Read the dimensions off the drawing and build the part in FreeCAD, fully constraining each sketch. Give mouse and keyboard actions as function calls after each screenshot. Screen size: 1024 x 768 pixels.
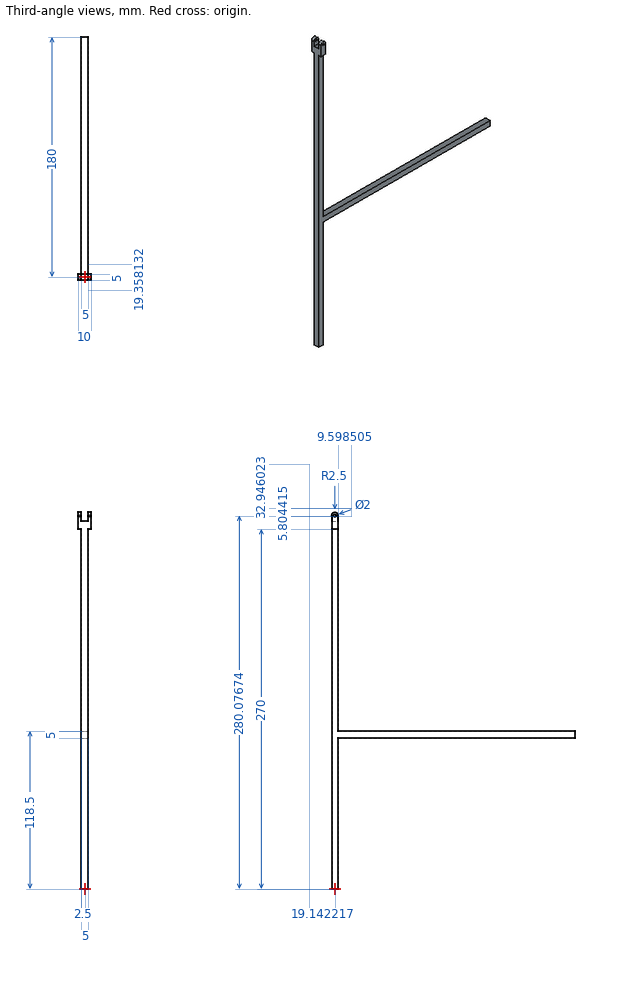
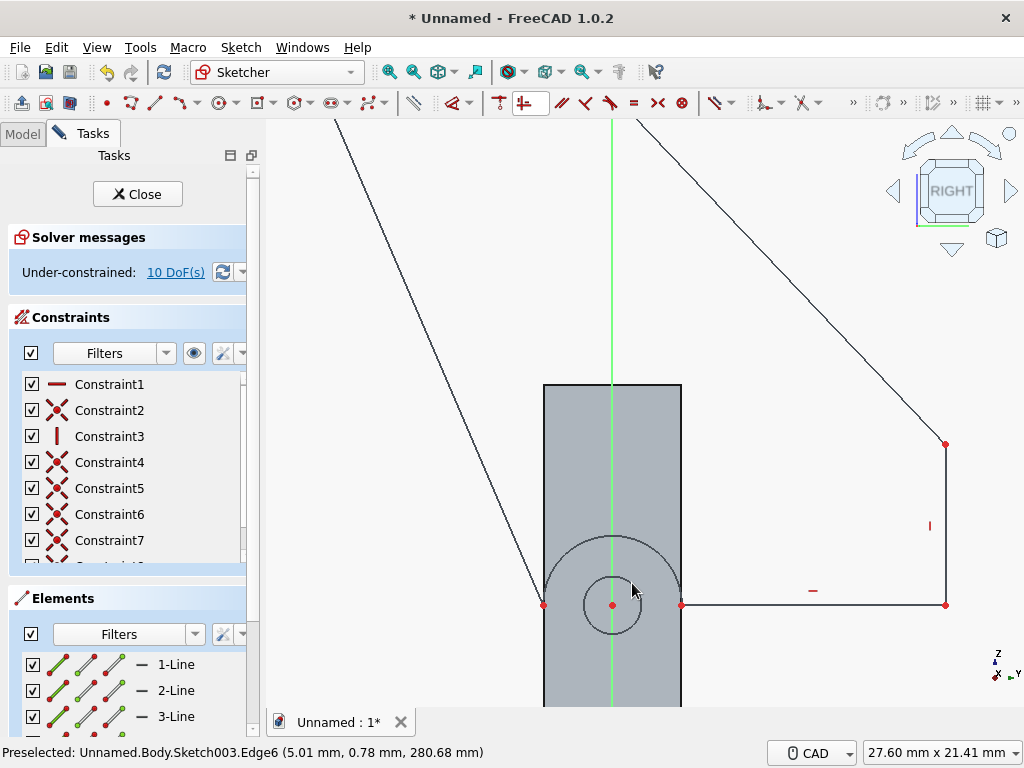
click(613, 605)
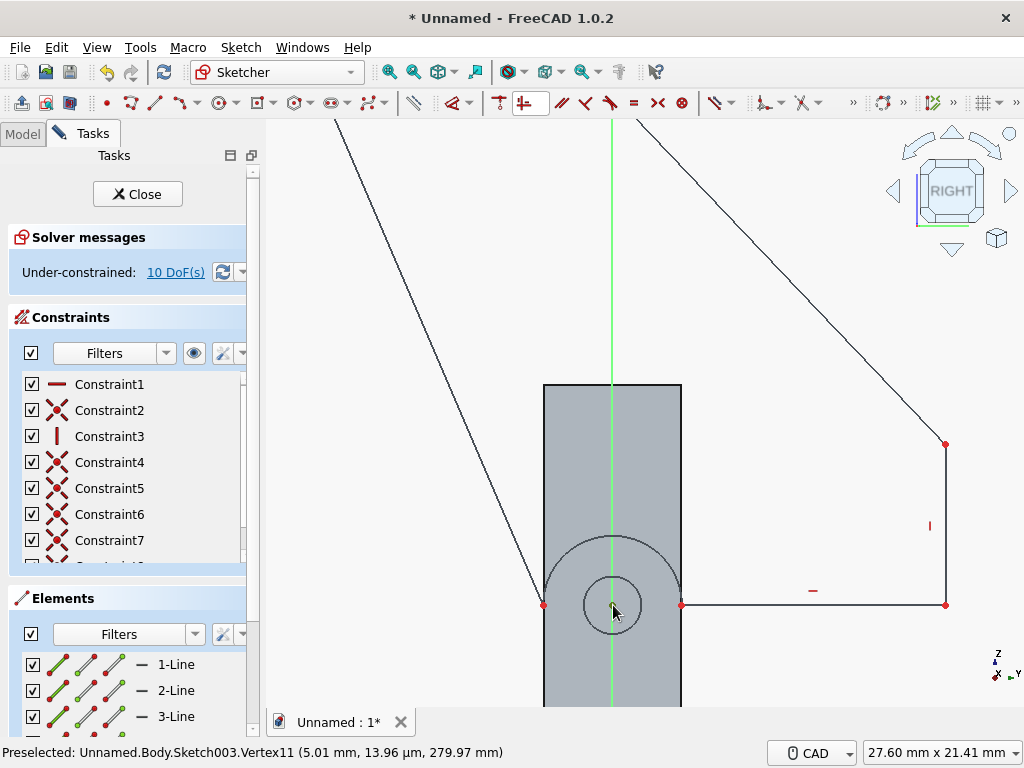
click(612, 489)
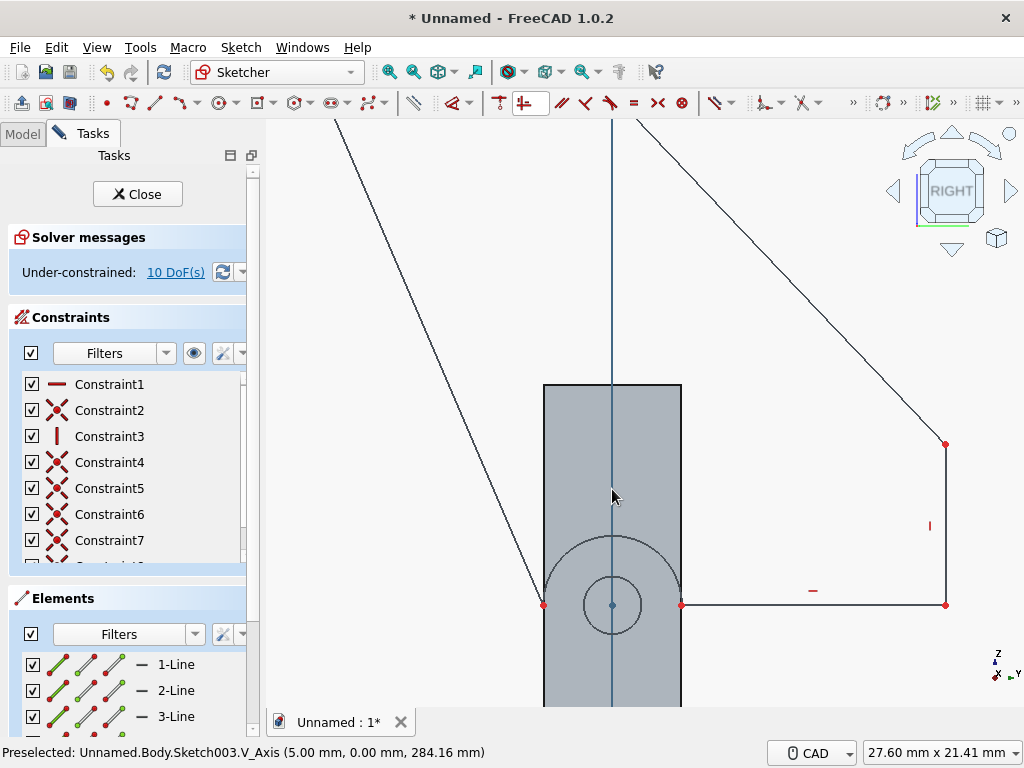
click(500, 104)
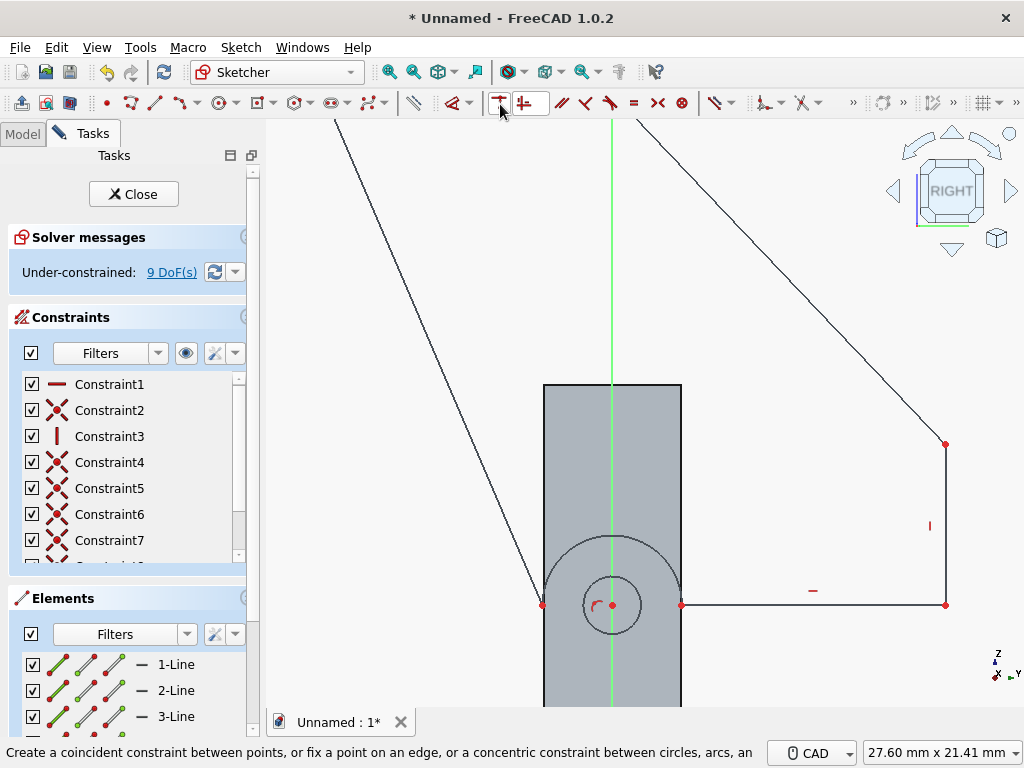
click(452, 104)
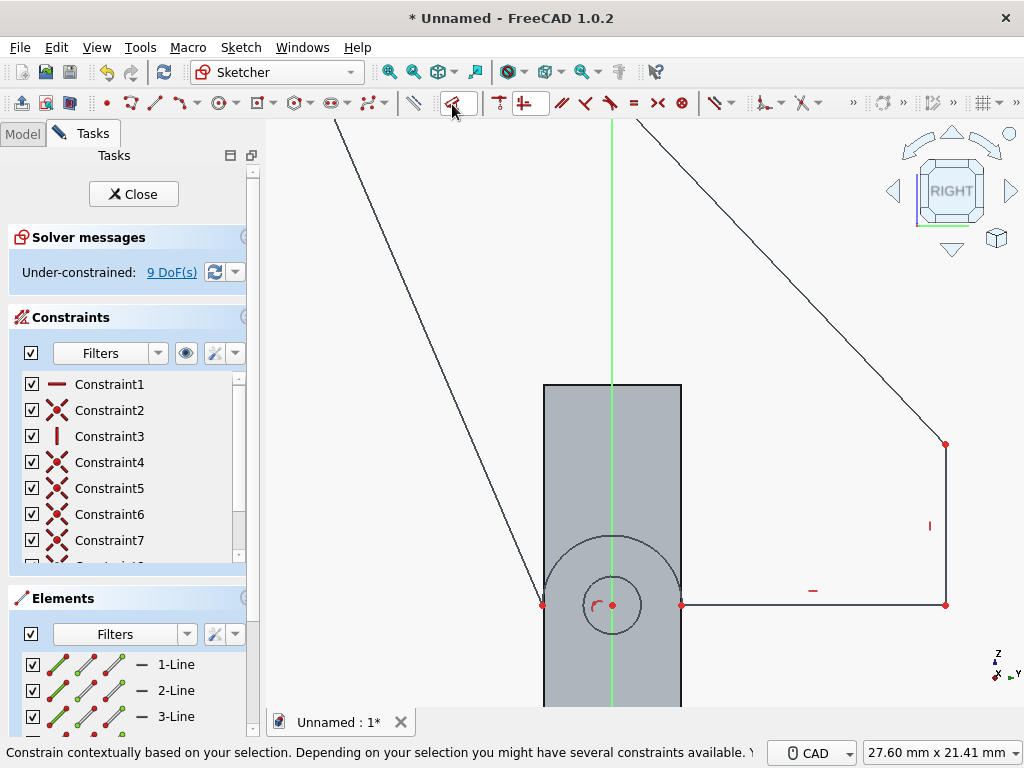
click(653, 549)
click(672, 523)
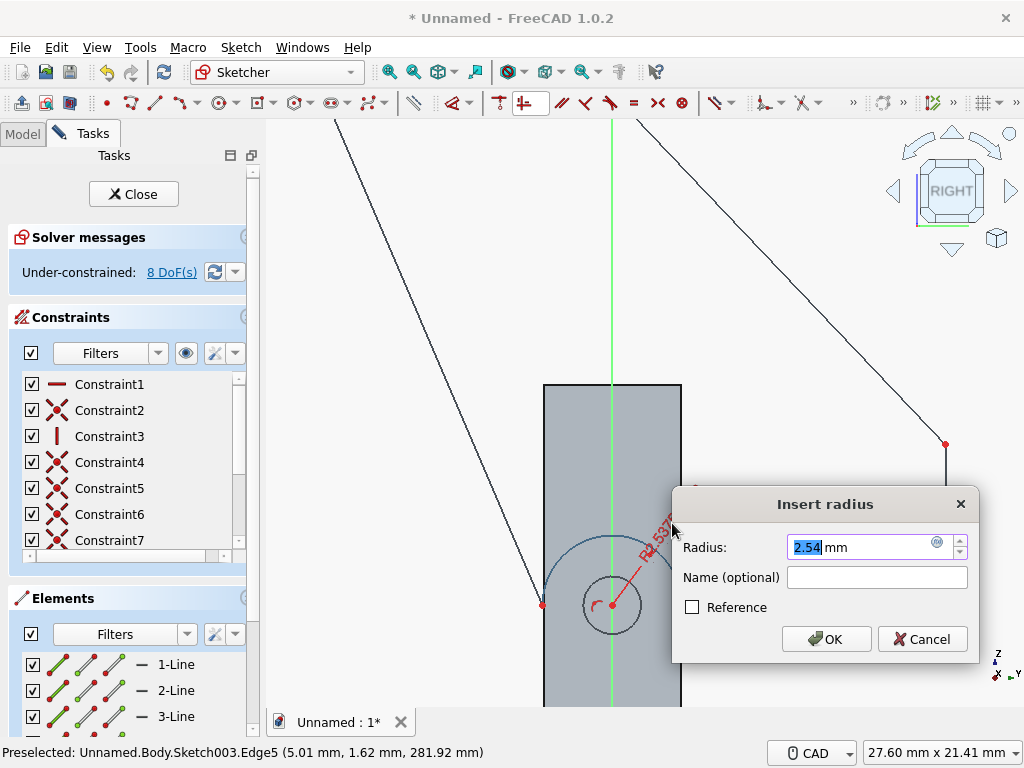
text(2.5)
key(Return)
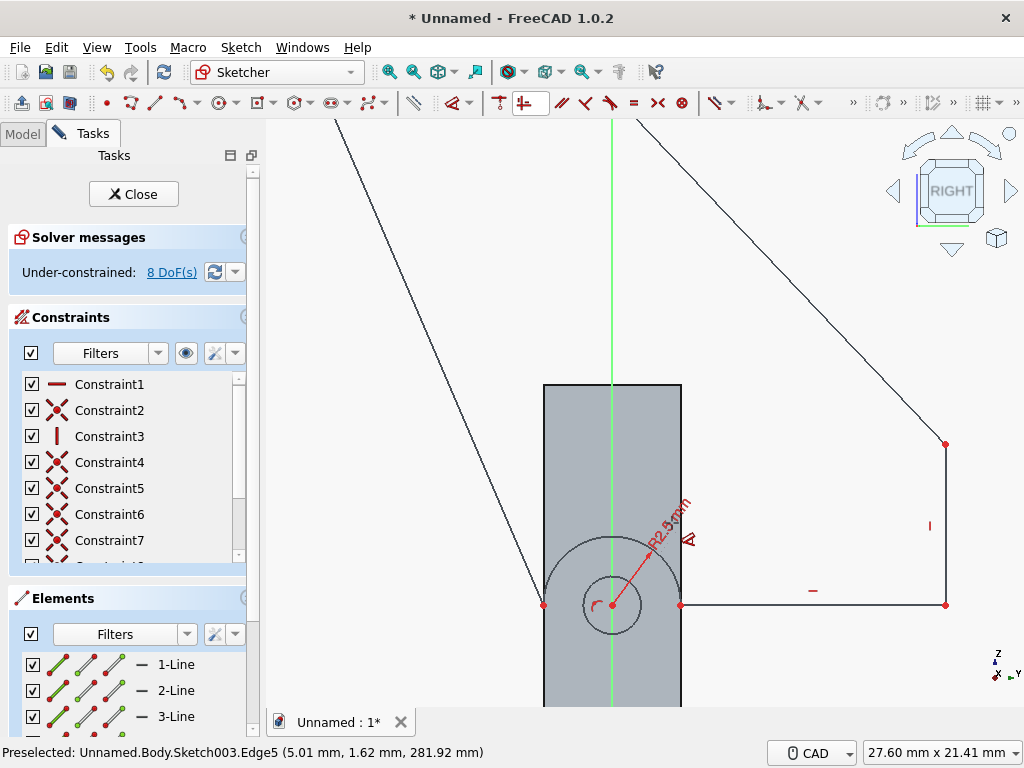
click(632, 585)
click(671, 617)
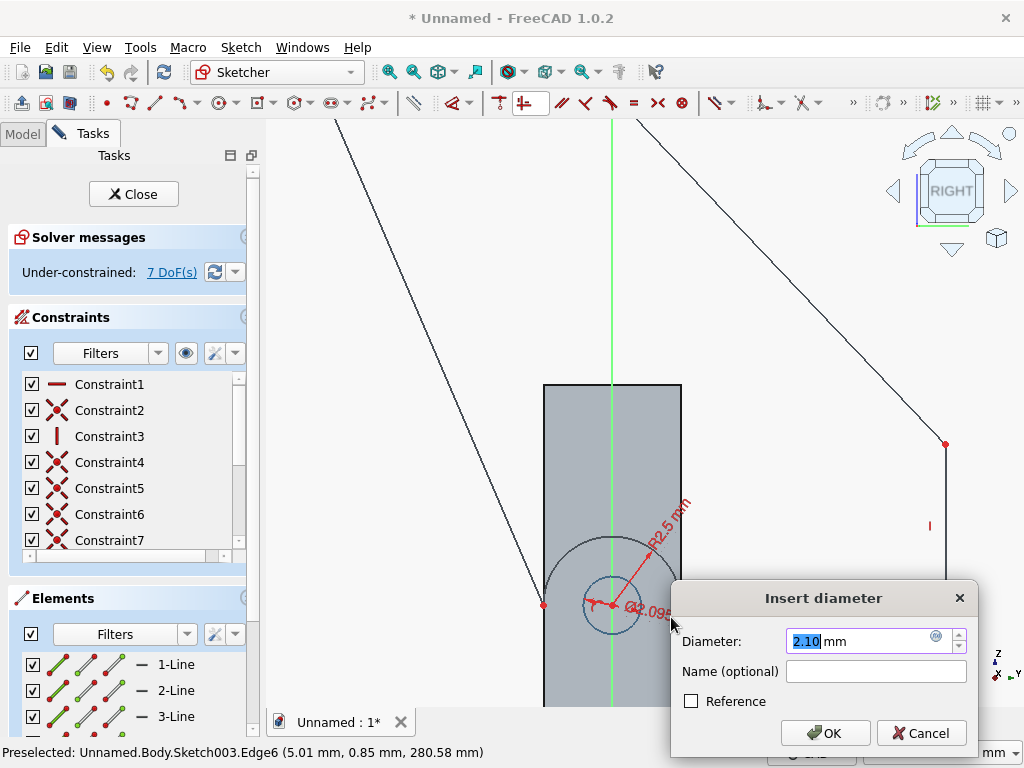
text(2)
key(Return)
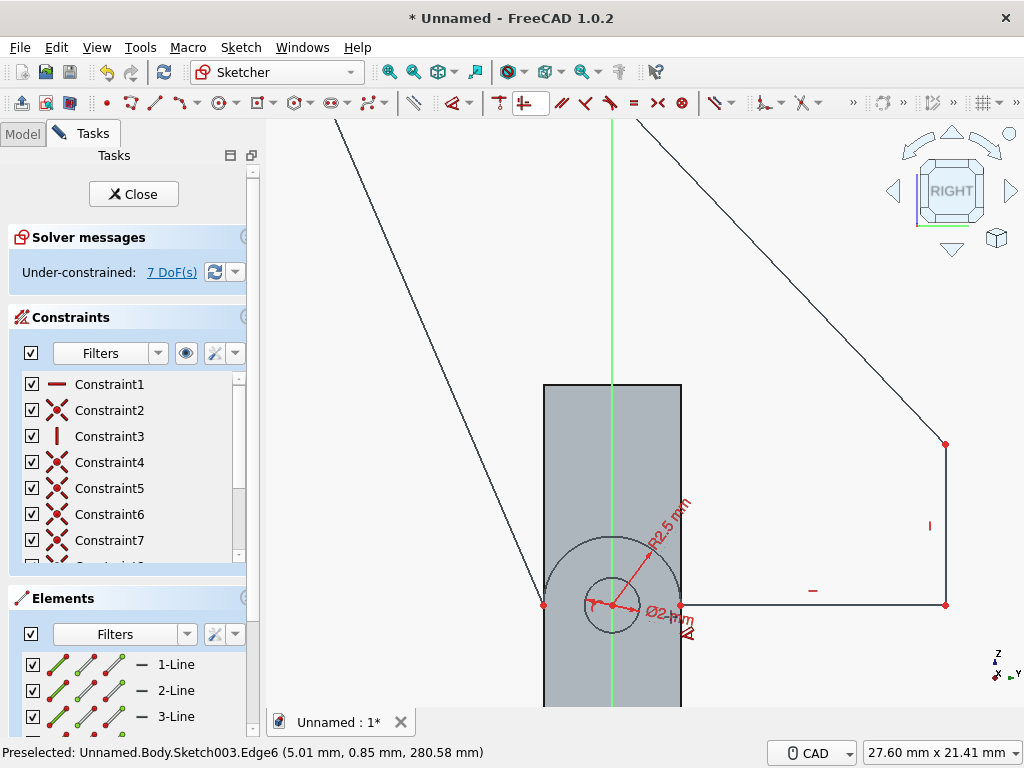
click(760, 605)
click(770, 639)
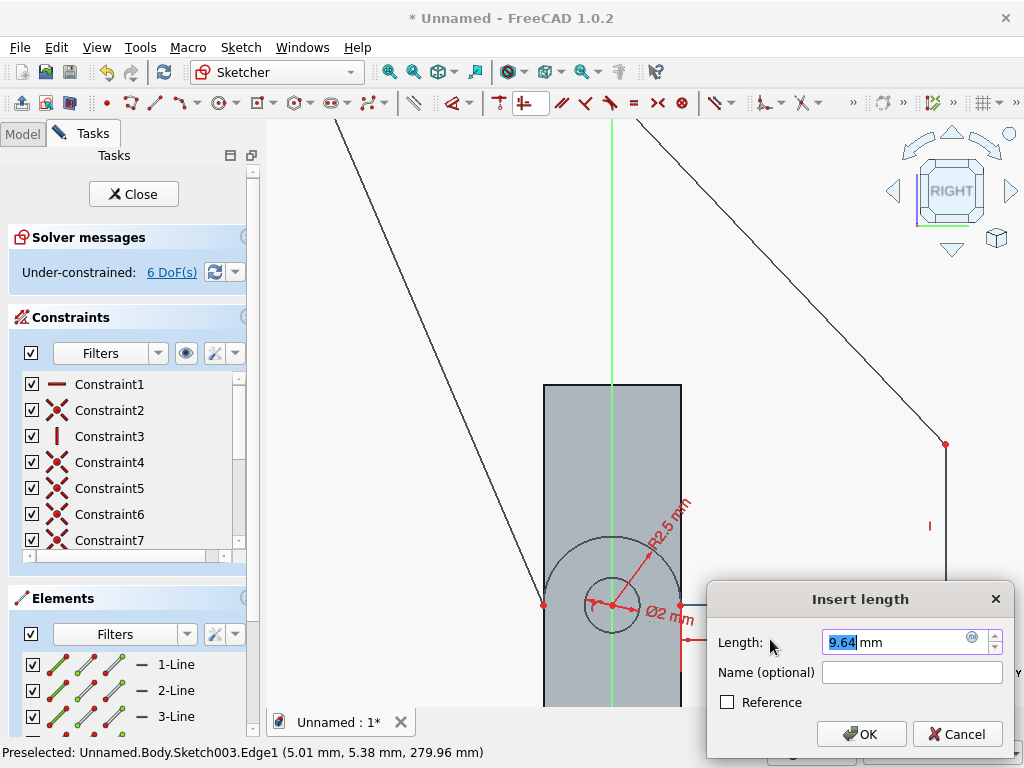
text(9.598505)
key(Return)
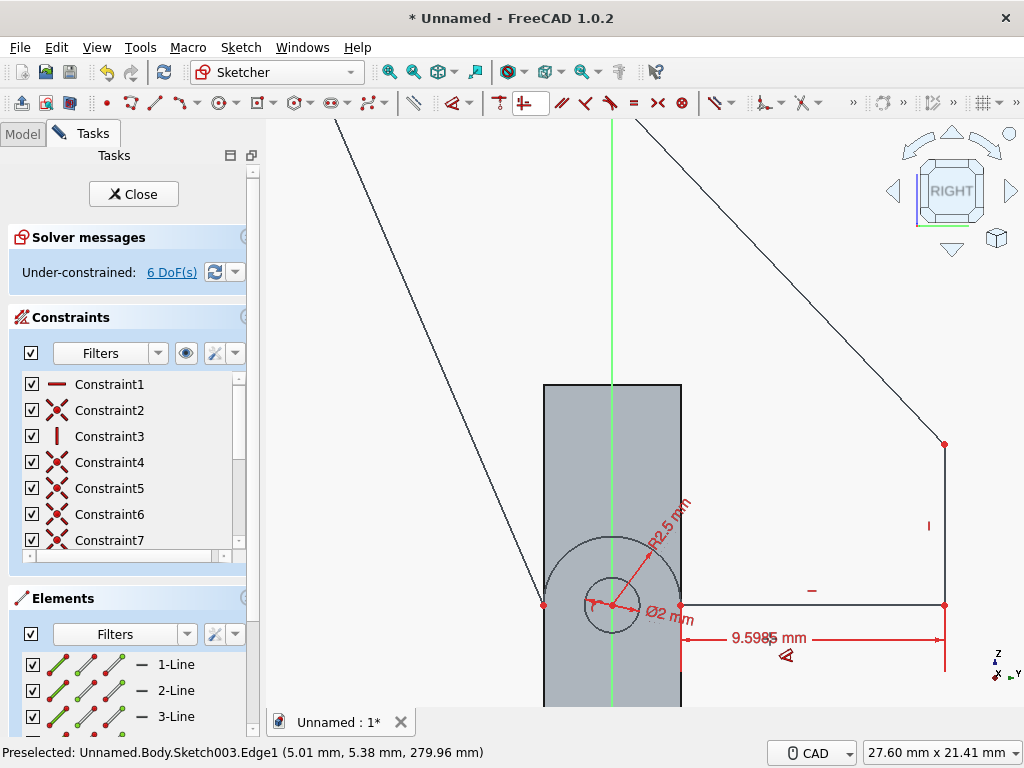
scroll(612, 605, down, 5)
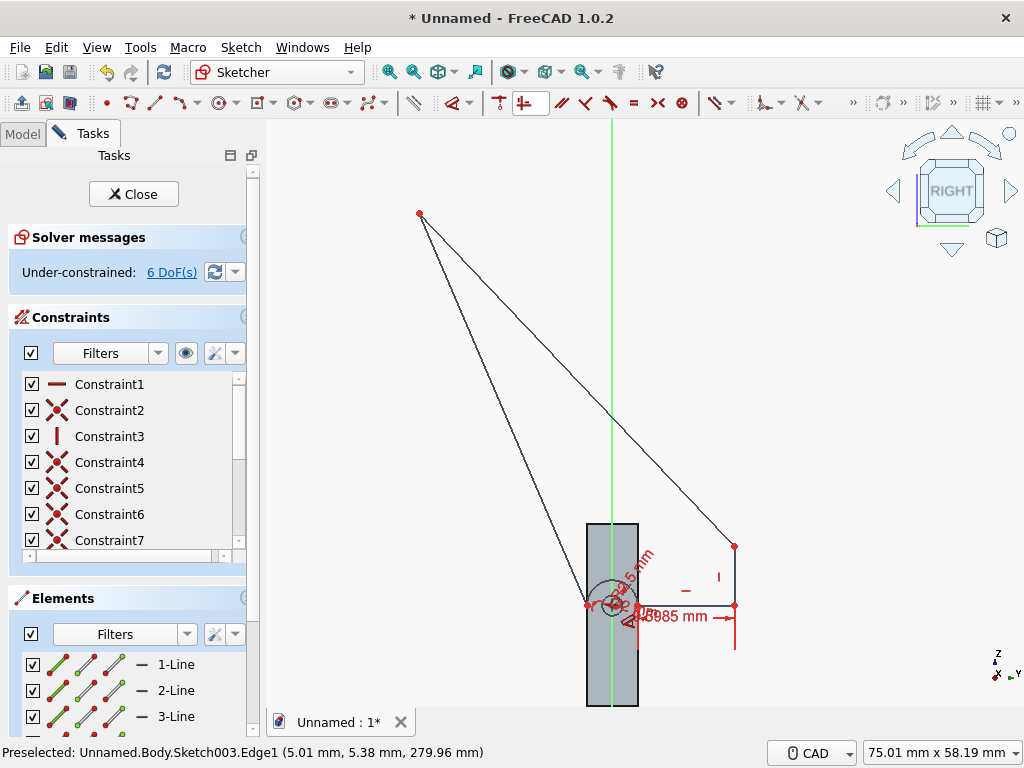
click(735, 588)
click(769, 576)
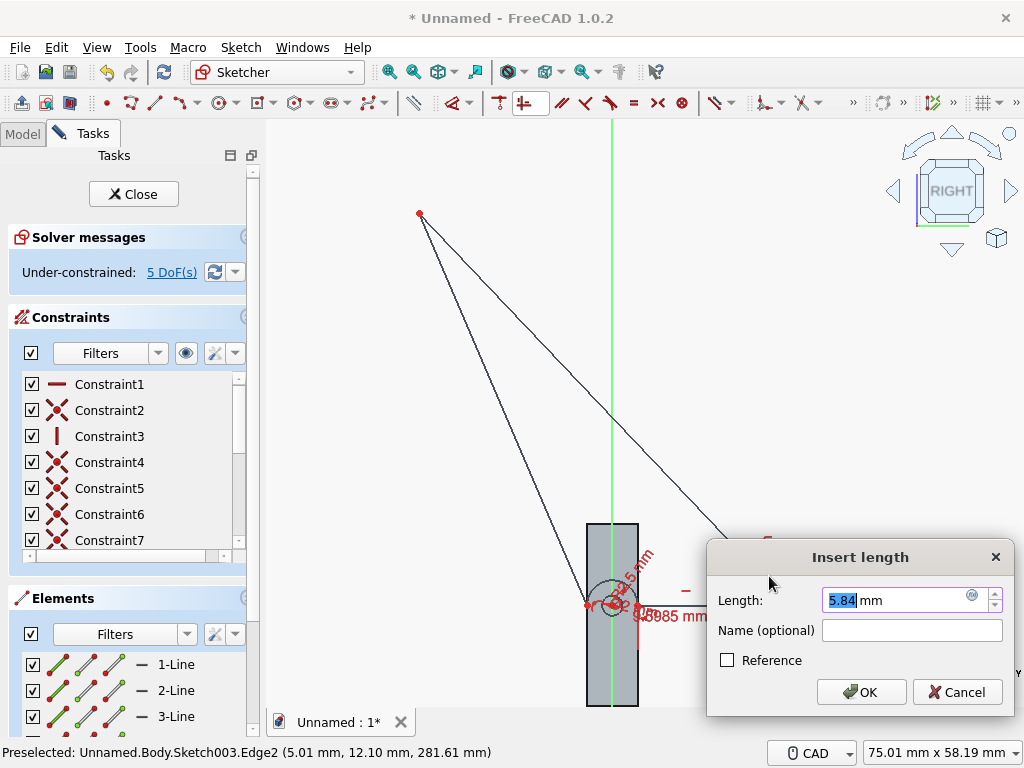
text(5.804415)
key(Return)